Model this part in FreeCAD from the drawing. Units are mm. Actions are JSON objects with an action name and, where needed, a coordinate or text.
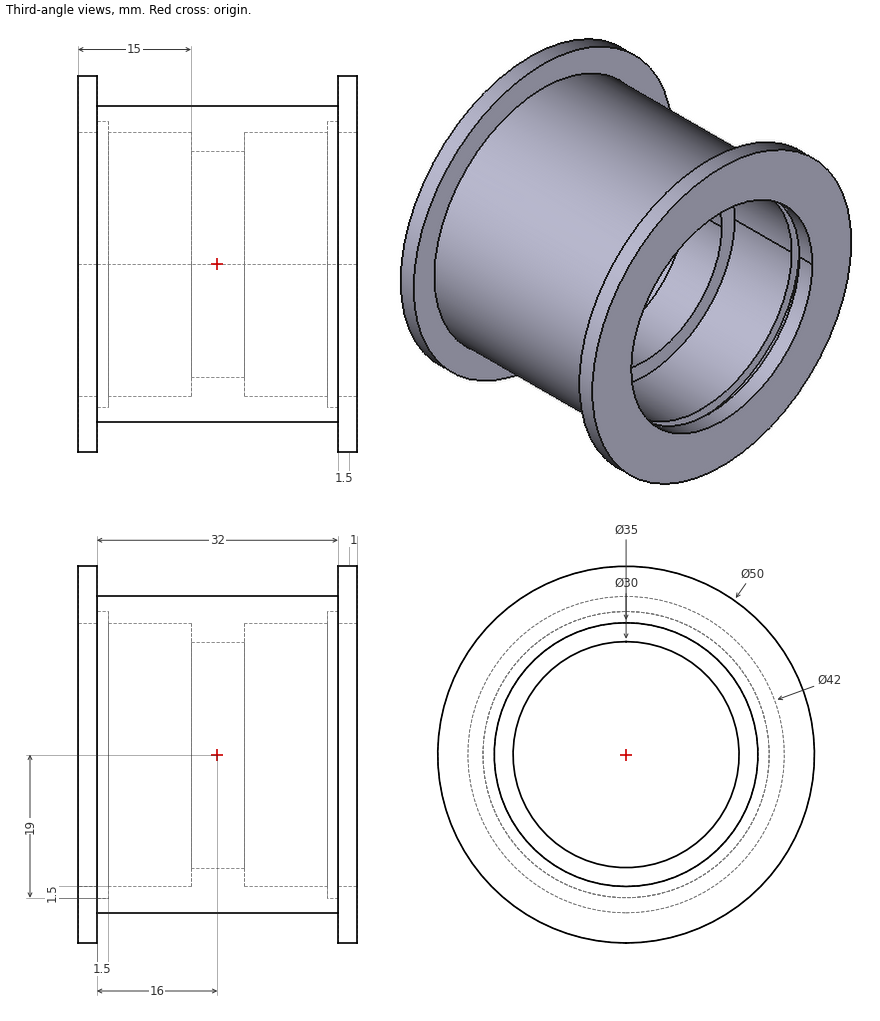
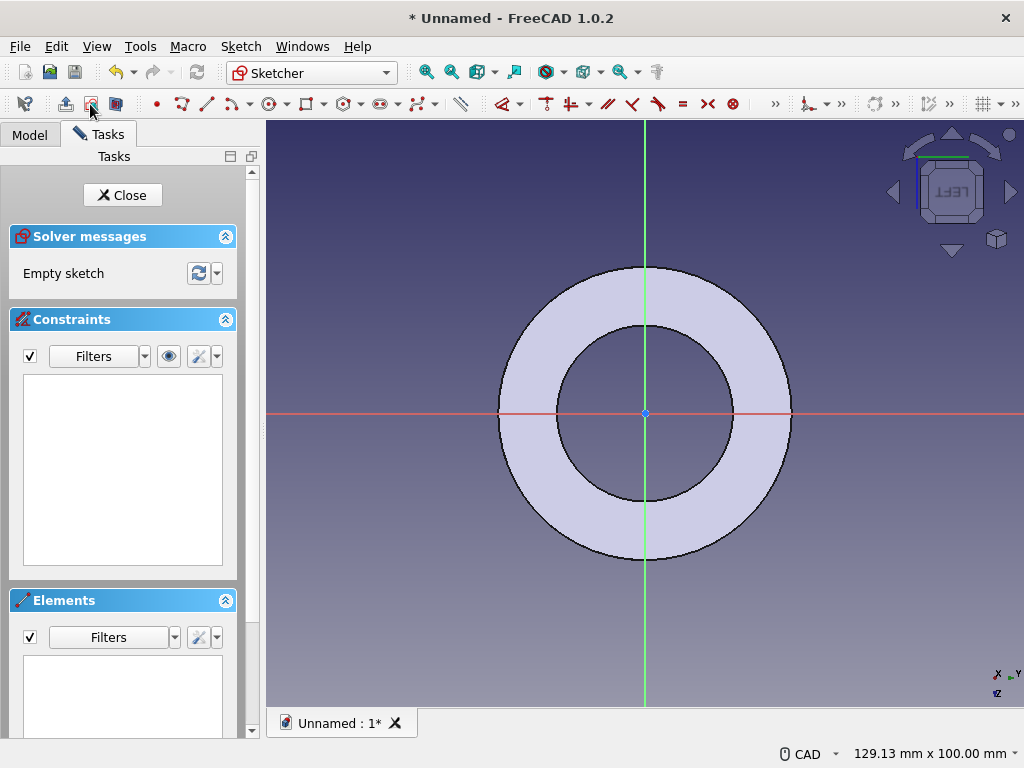
{"action": "scroll", "coordinate": [728, 413], "scroll_direction": "up", "scroll_amount": 3}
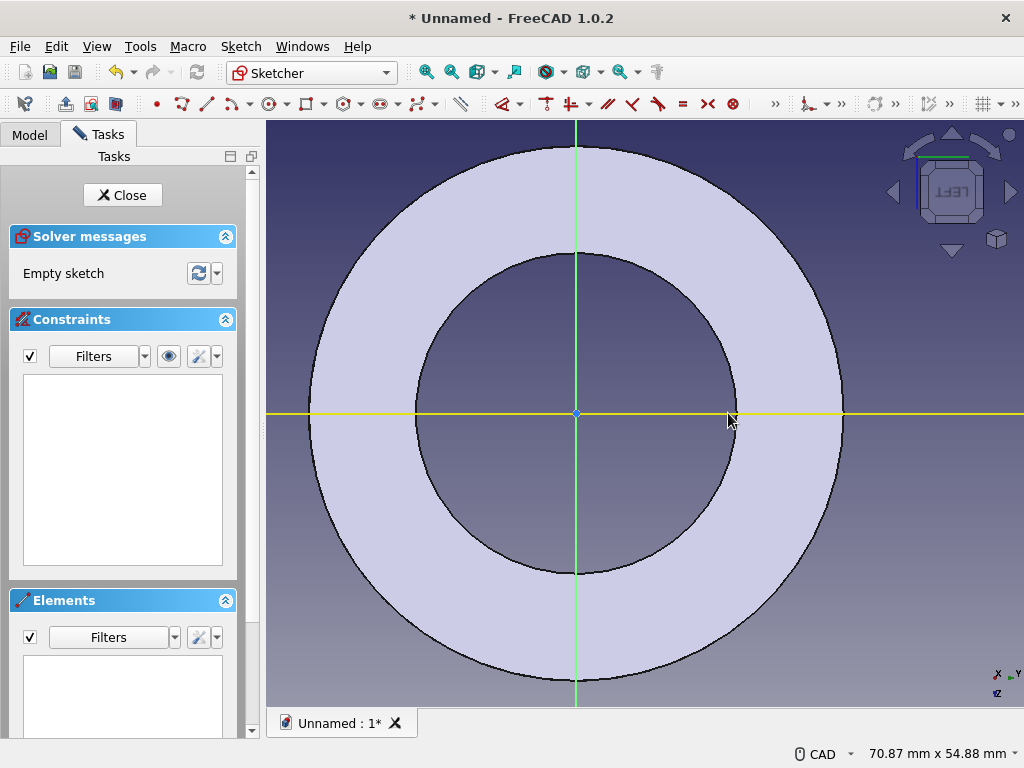
{"action": "left_click", "coordinate": [268, 104]}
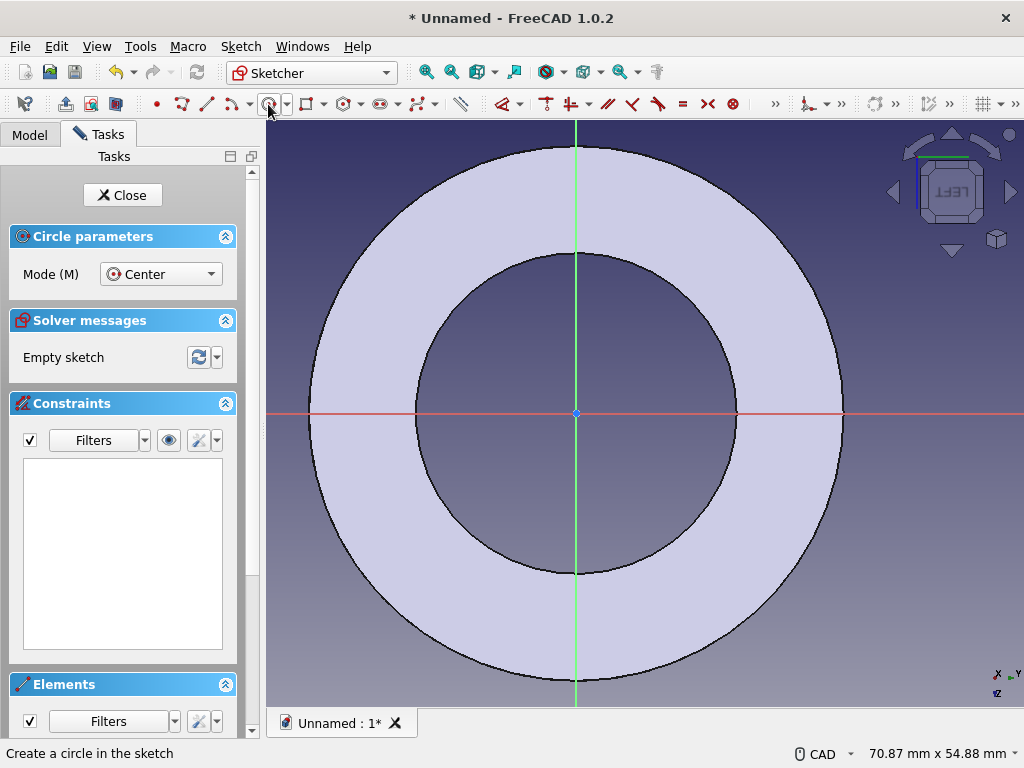
{"action": "left_click", "coordinate": [576, 413]}
{"action": "mouse_move", "coordinate": [709, 281]}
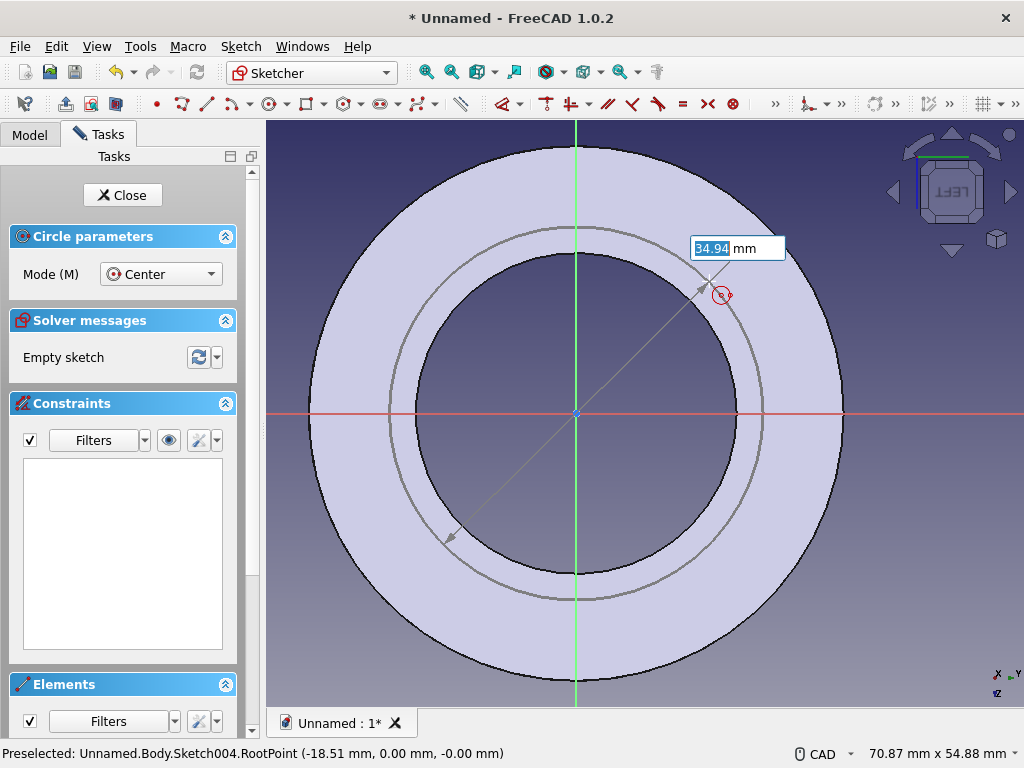
{"action": "type", "text": "35"}
{"action": "key", "text": "Return"}
{"action": "key", "text": "Escape"}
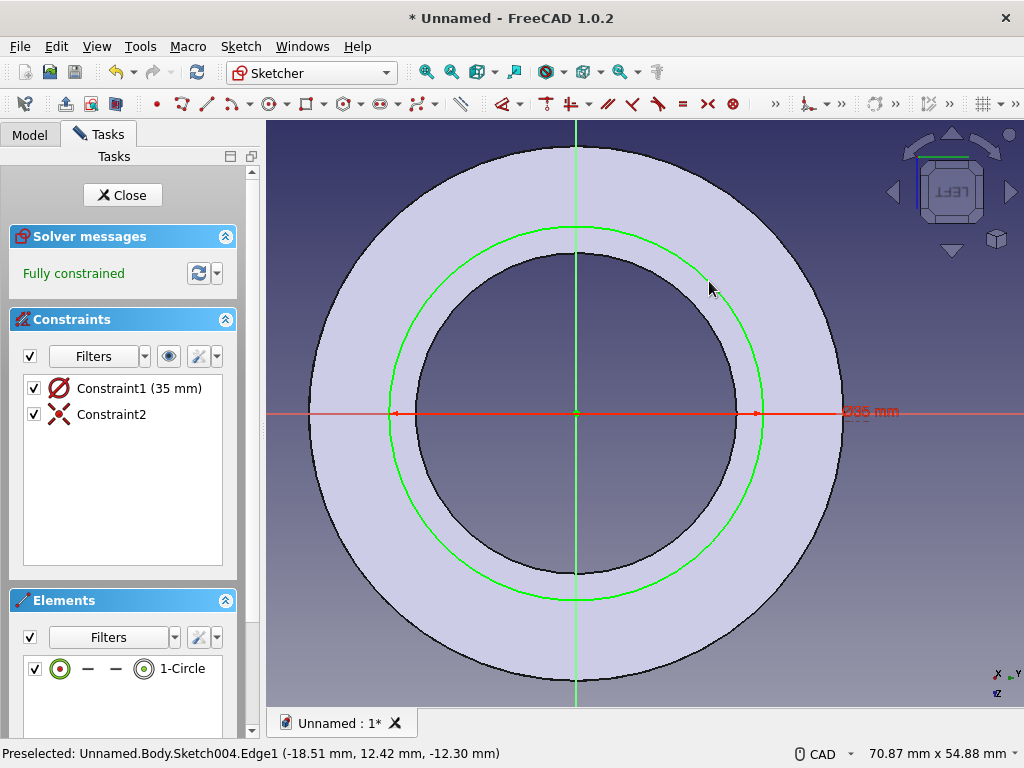
{"action": "left_click", "coordinate": [123, 195]}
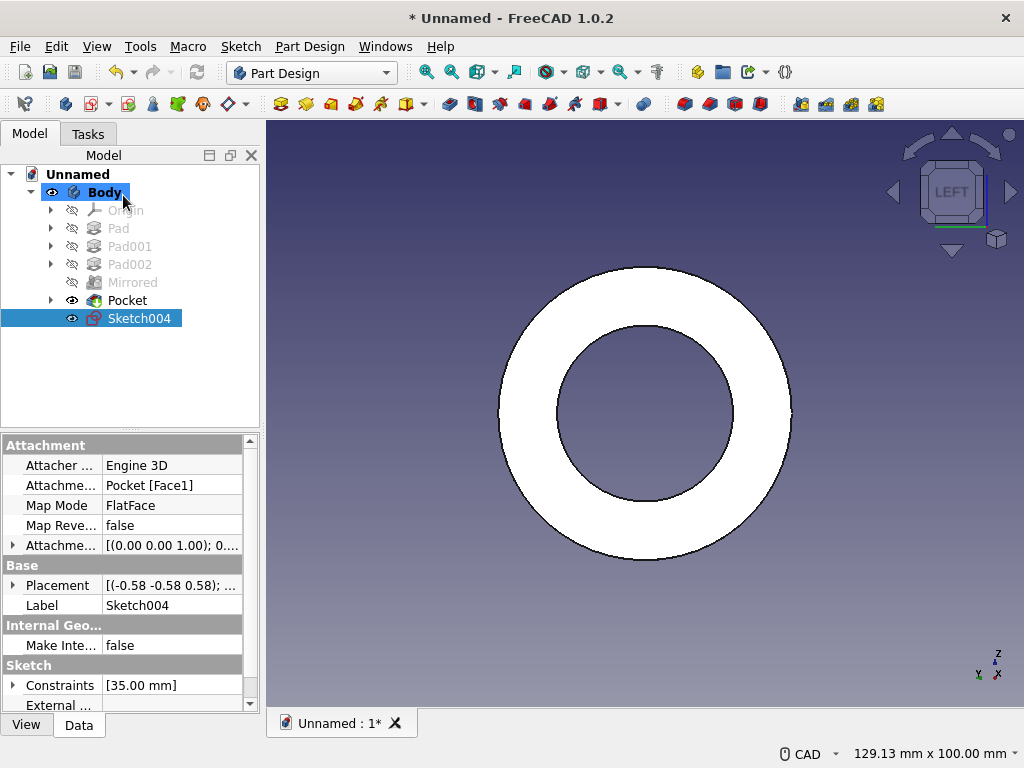
{"action": "left_click", "coordinate": [450, 104]}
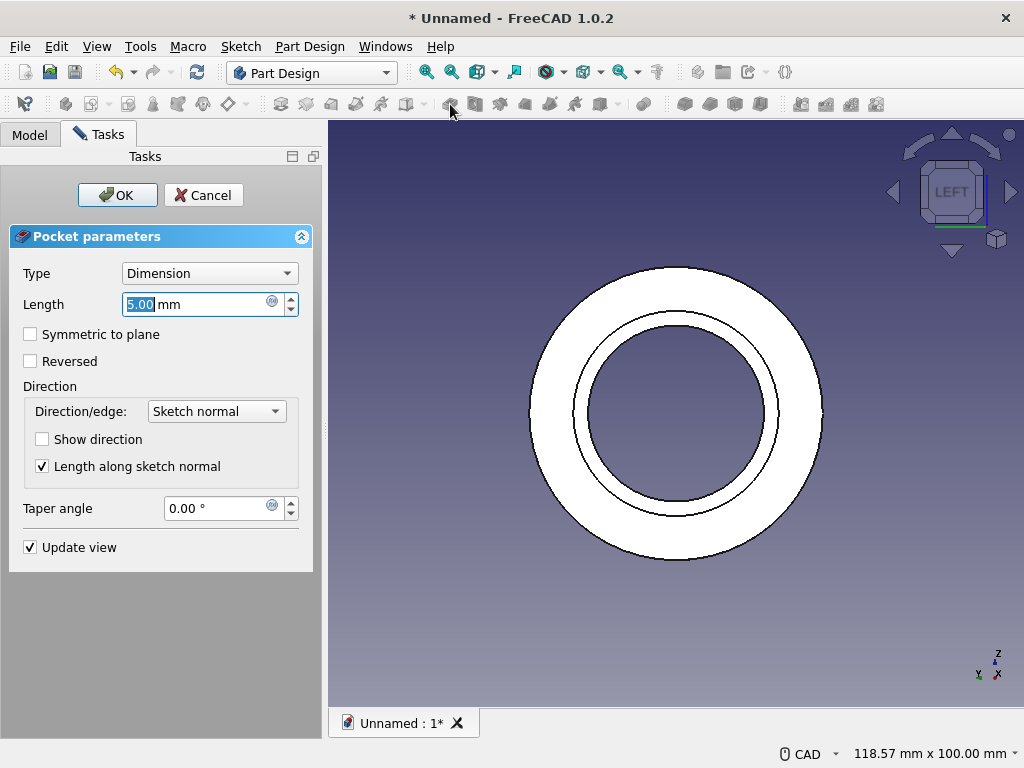
{"action": "type", "text": "15"}
{"action": "key", "text": "Tab"}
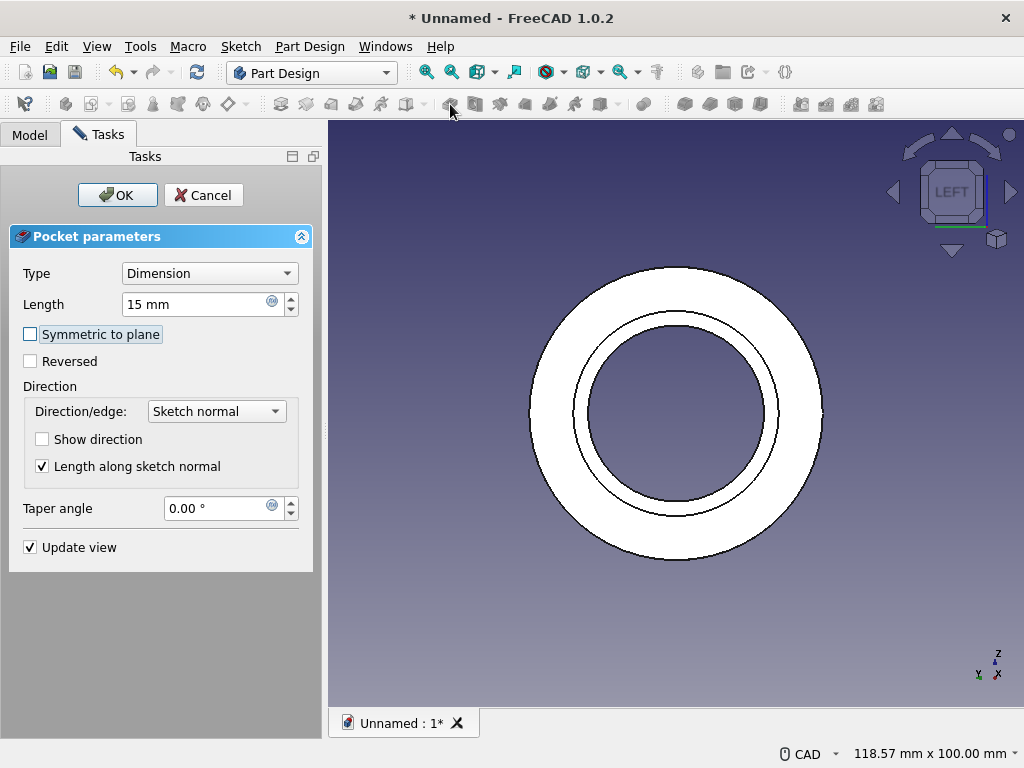
{"action": "left_click", "coordinate": [118, 195]}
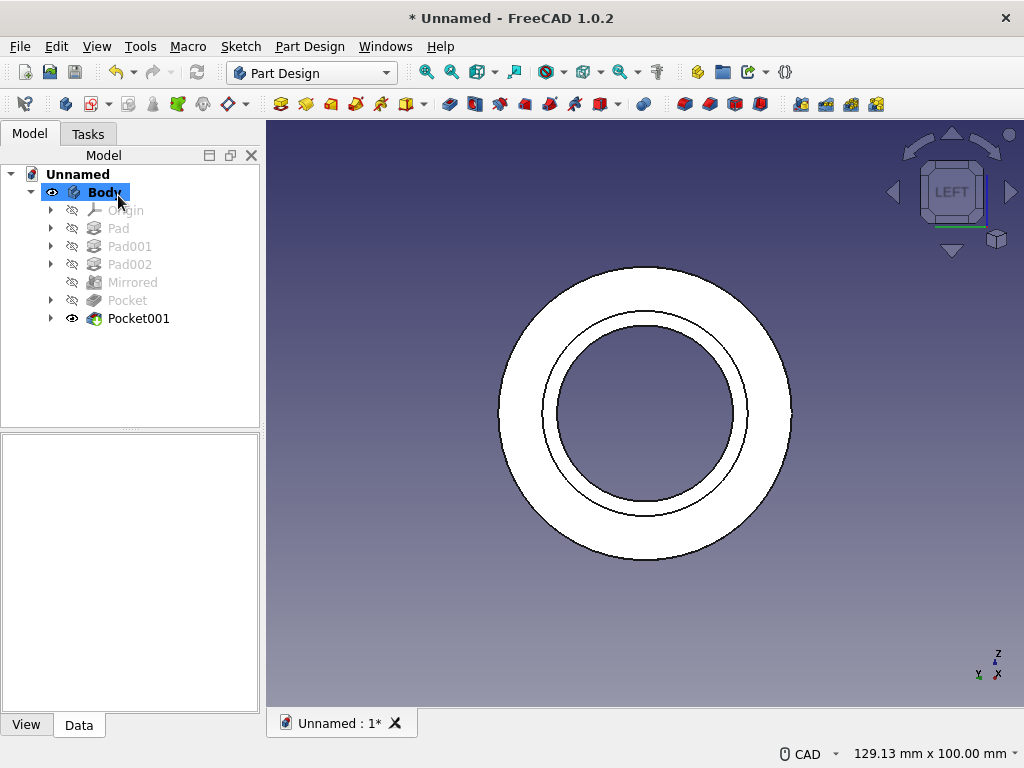
{"action": "left_click", "coordinate": [90, 104]}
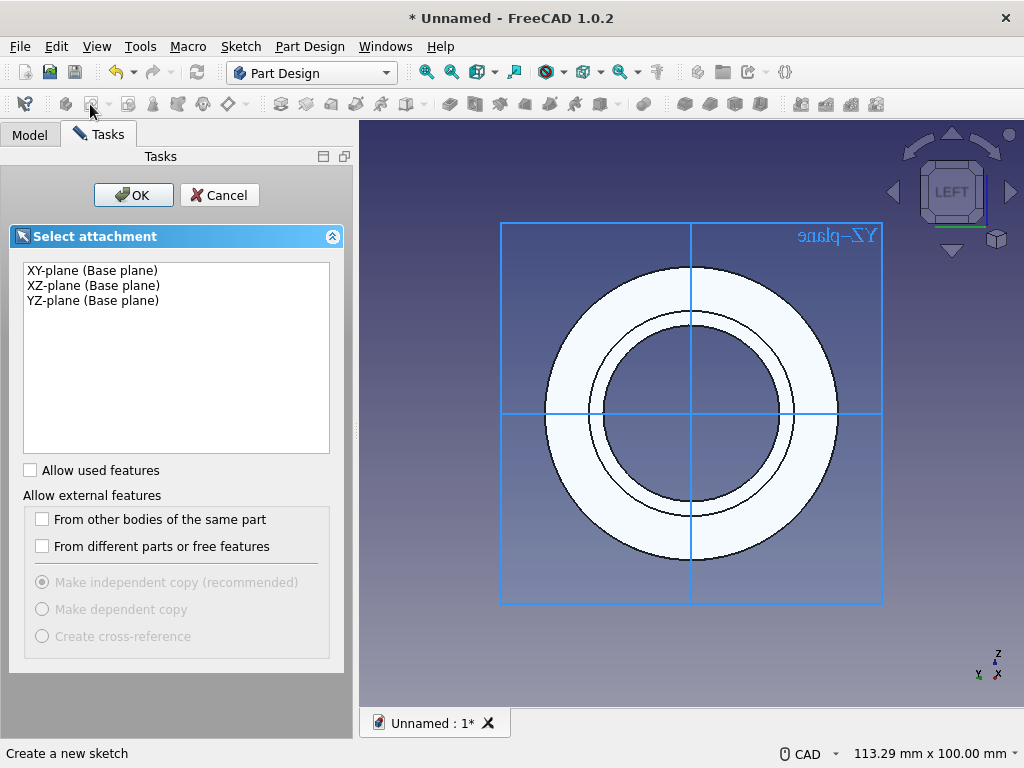
{"action": "left_click", "coordinate": [84, 286]}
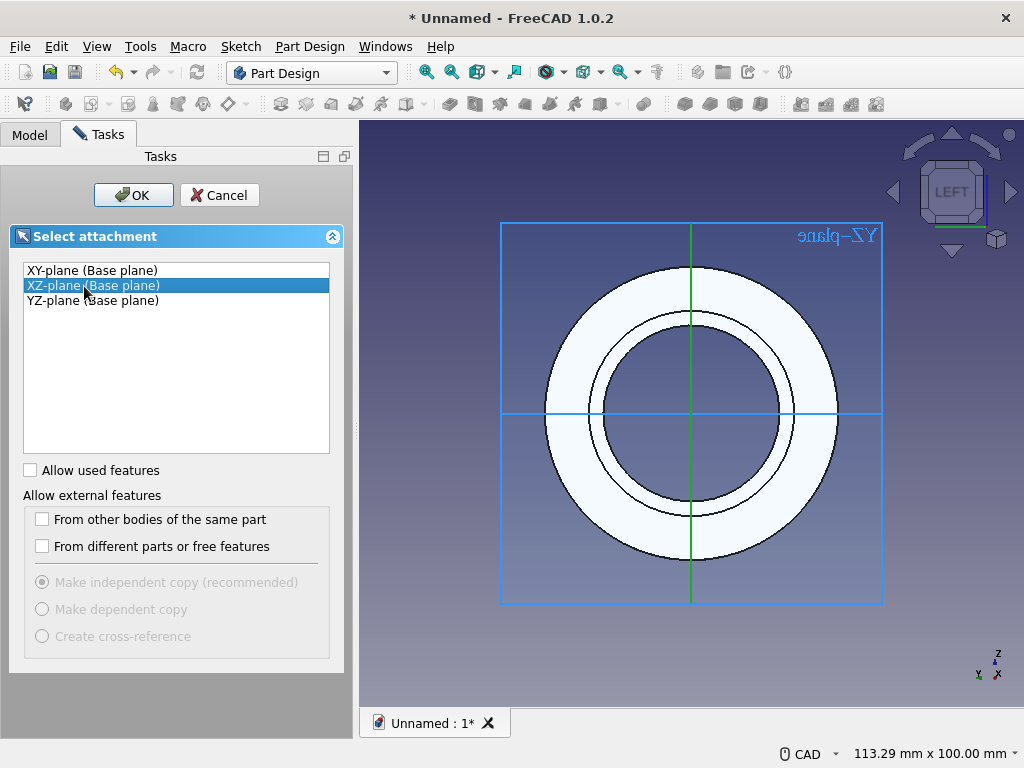
{"action": "left_click", "coordinate": [134, 195]}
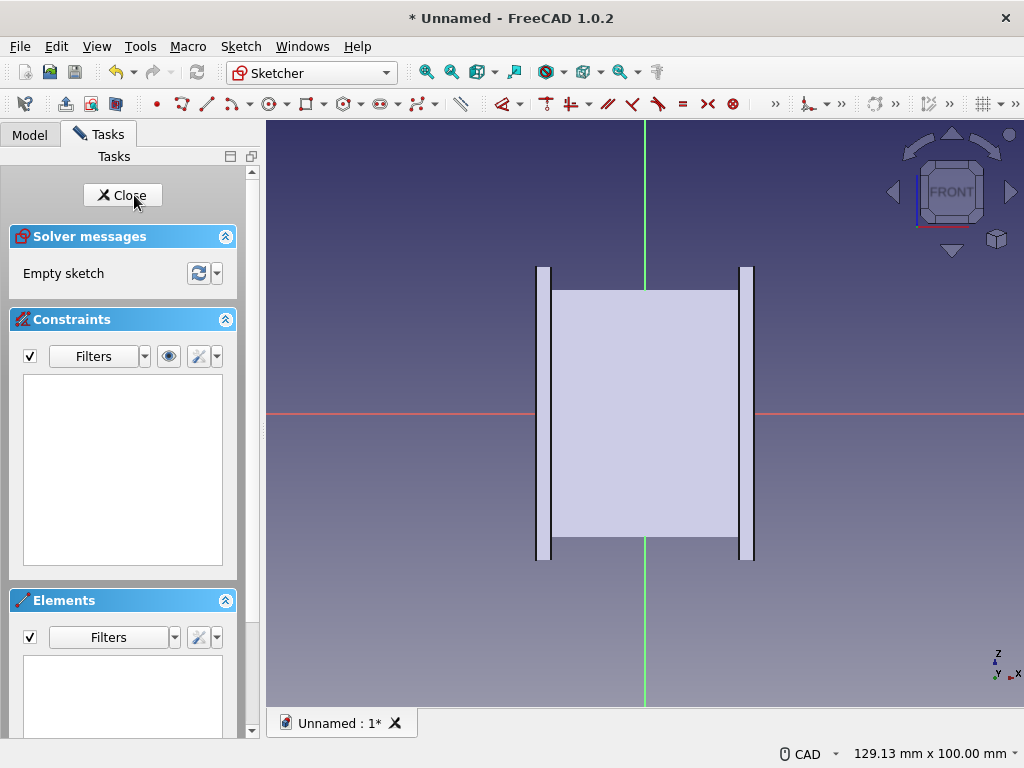
{"action": "key", "text": "q s"}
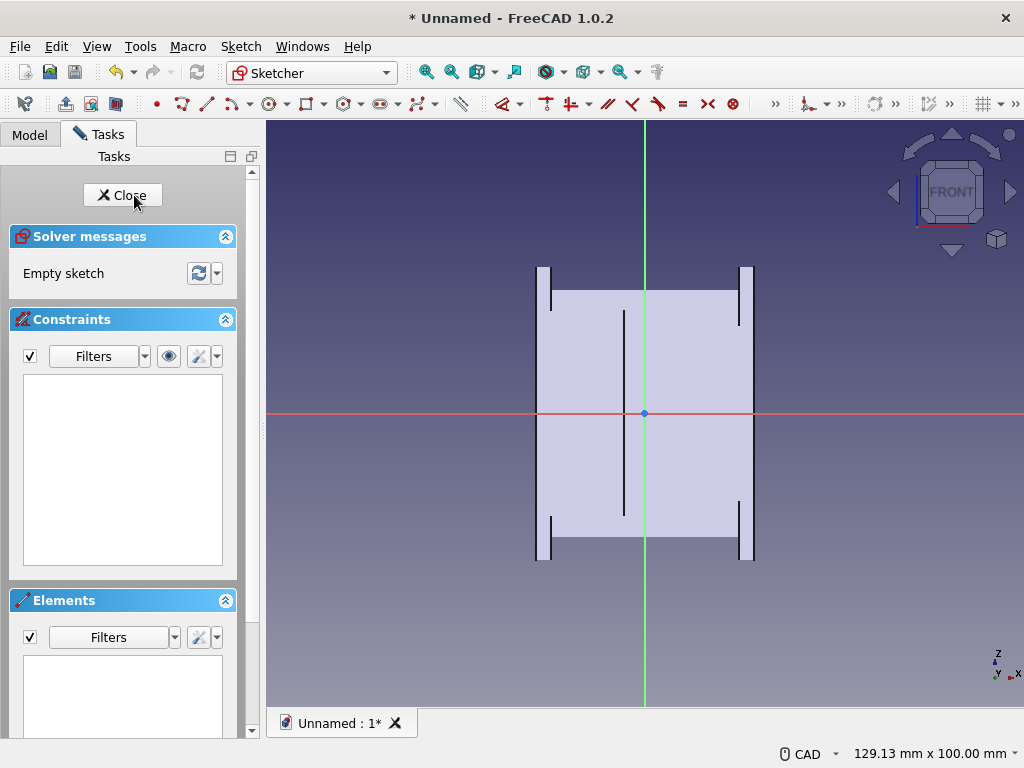
{"action": "scroll", "coordinate": [554, 526], "scroll_direction": "up", "scroll_amount": 15}